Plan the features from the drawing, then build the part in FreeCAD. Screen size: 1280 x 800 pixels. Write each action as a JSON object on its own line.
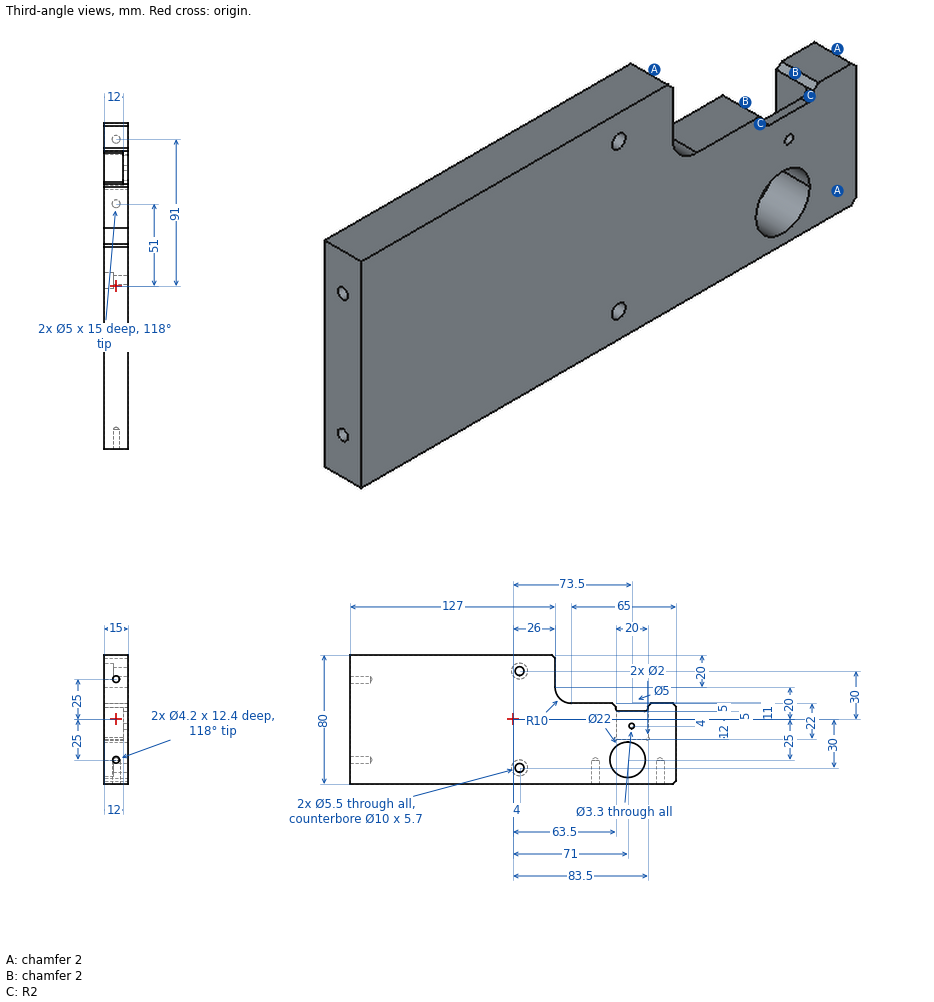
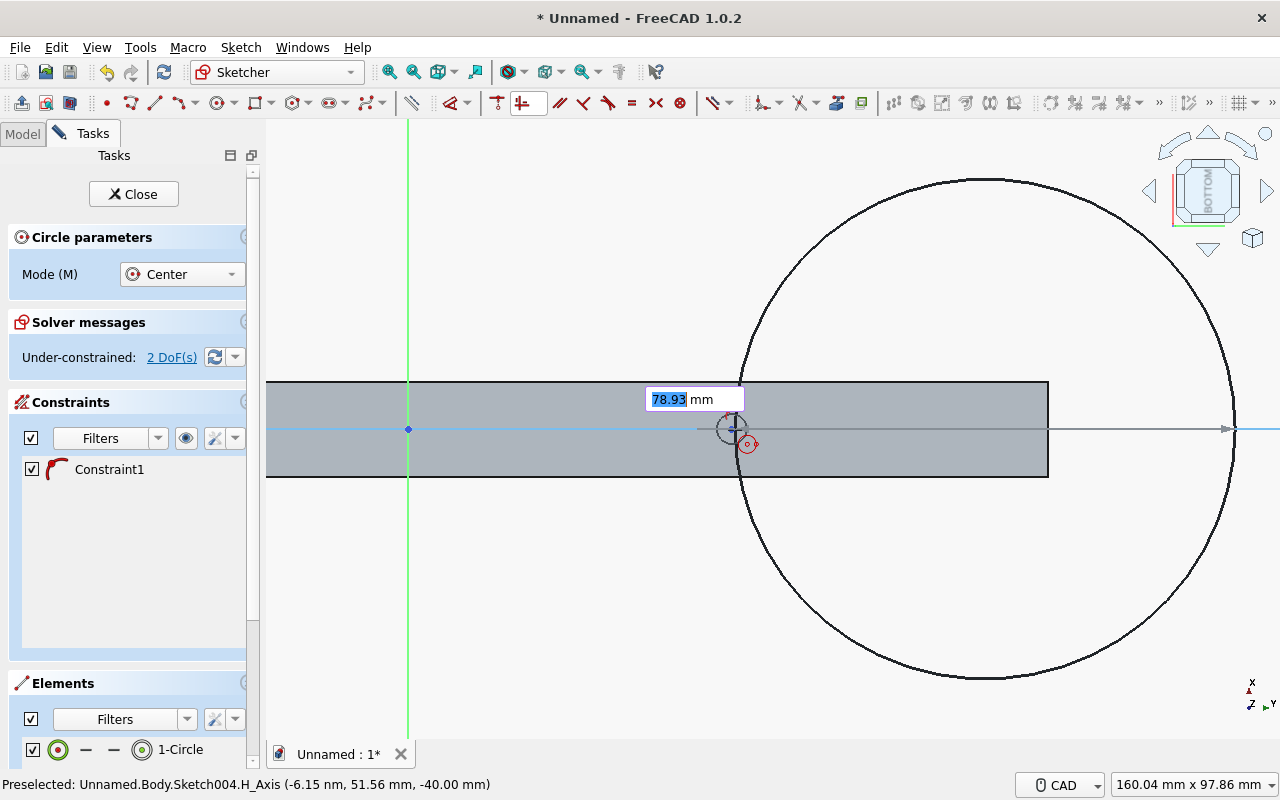
{"action": "scroll", "coordinate": [996, 418], "scroll_direction": "up", "scroll_amount": 2}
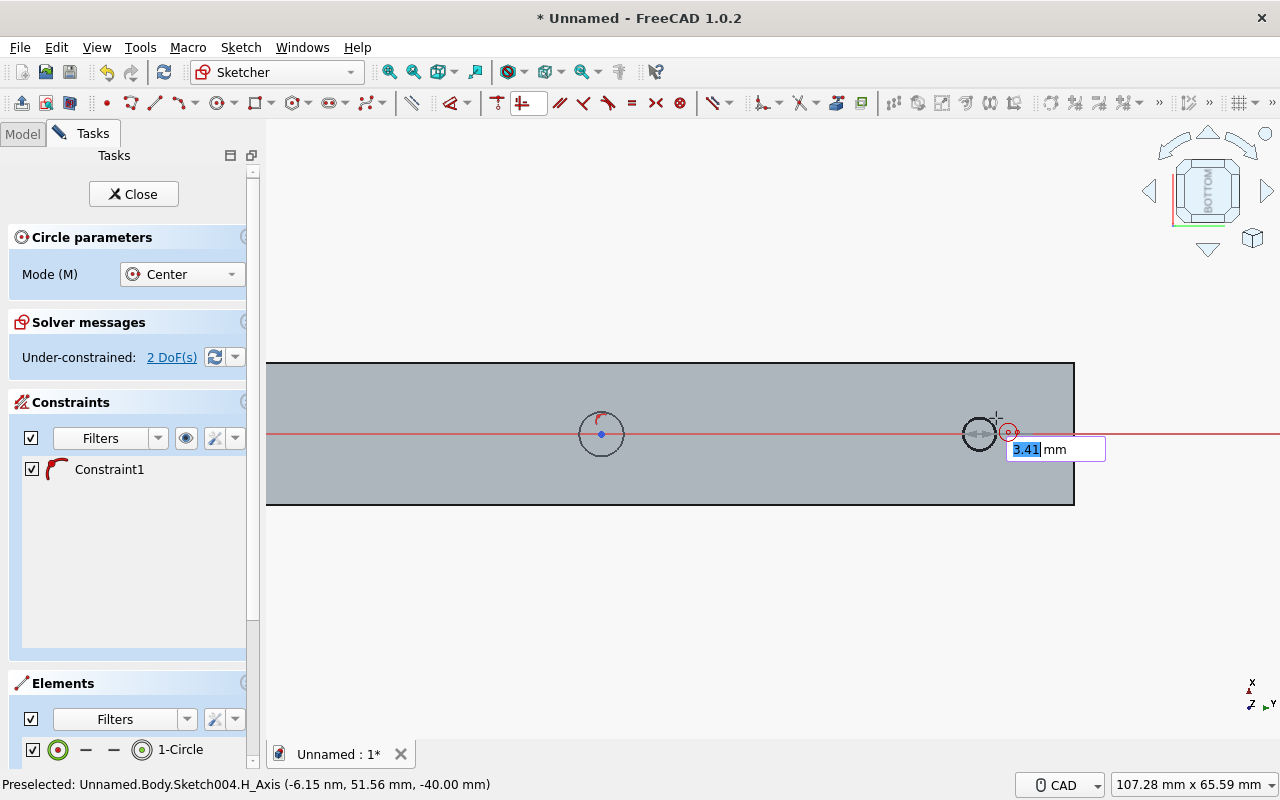
{"action": "left_click", "coordinate": [996, 418]}
{"action": "key", "text": "Escape"}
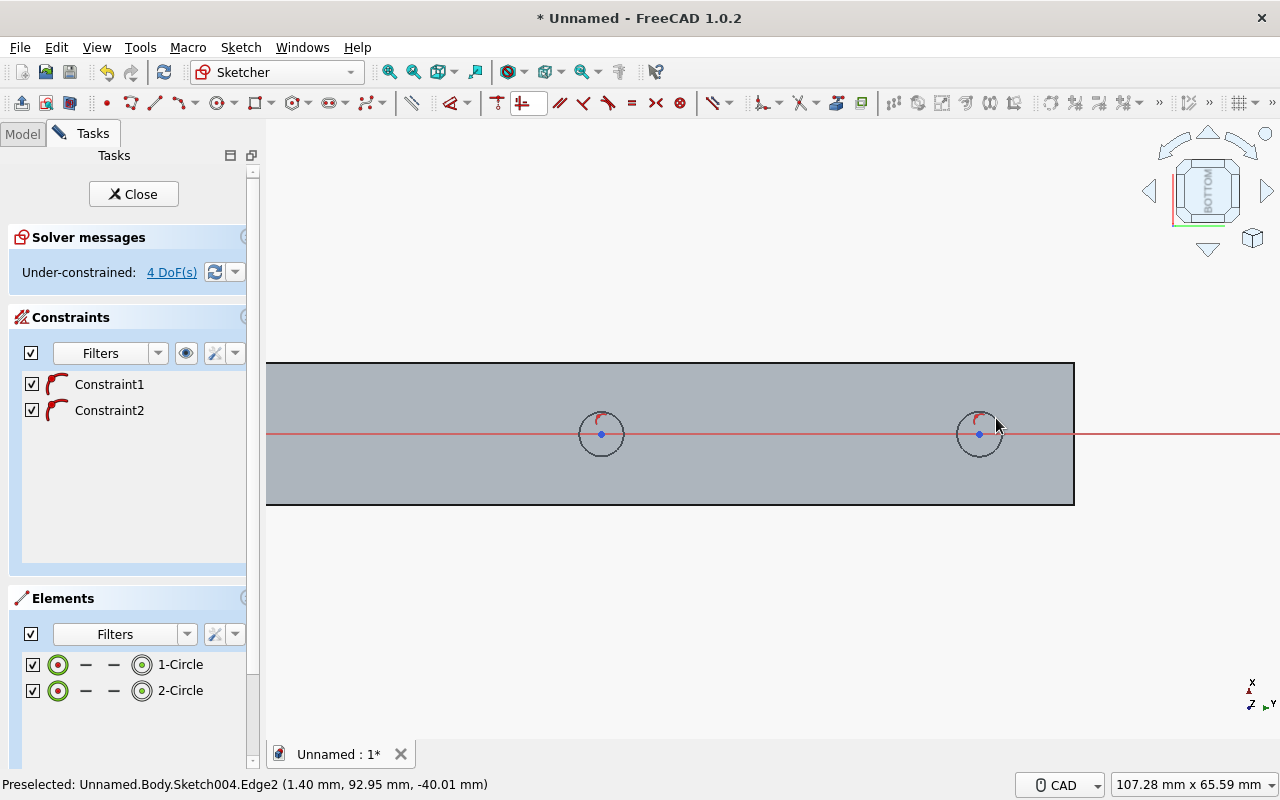
{"action": "left_click", "coordinate": [617, 419]}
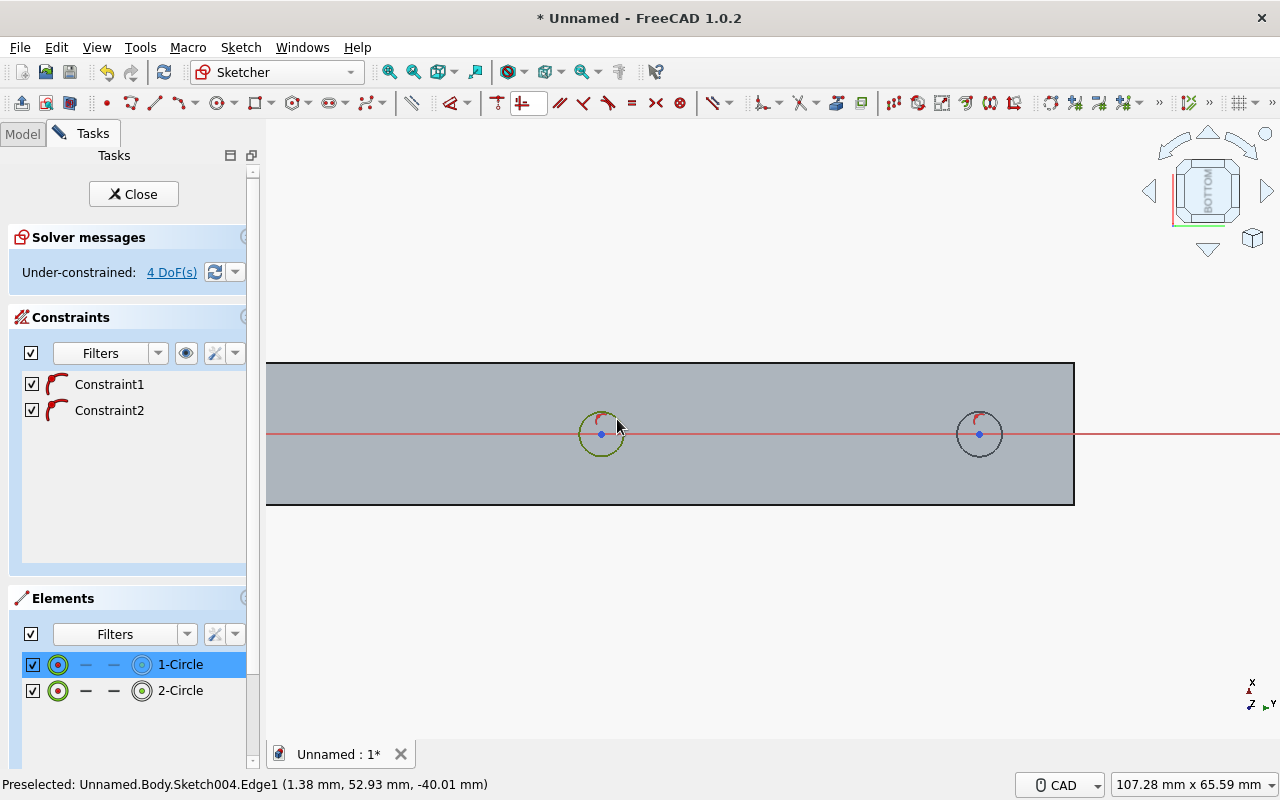
{"action": "left_click", "coordinate": [995, 418]}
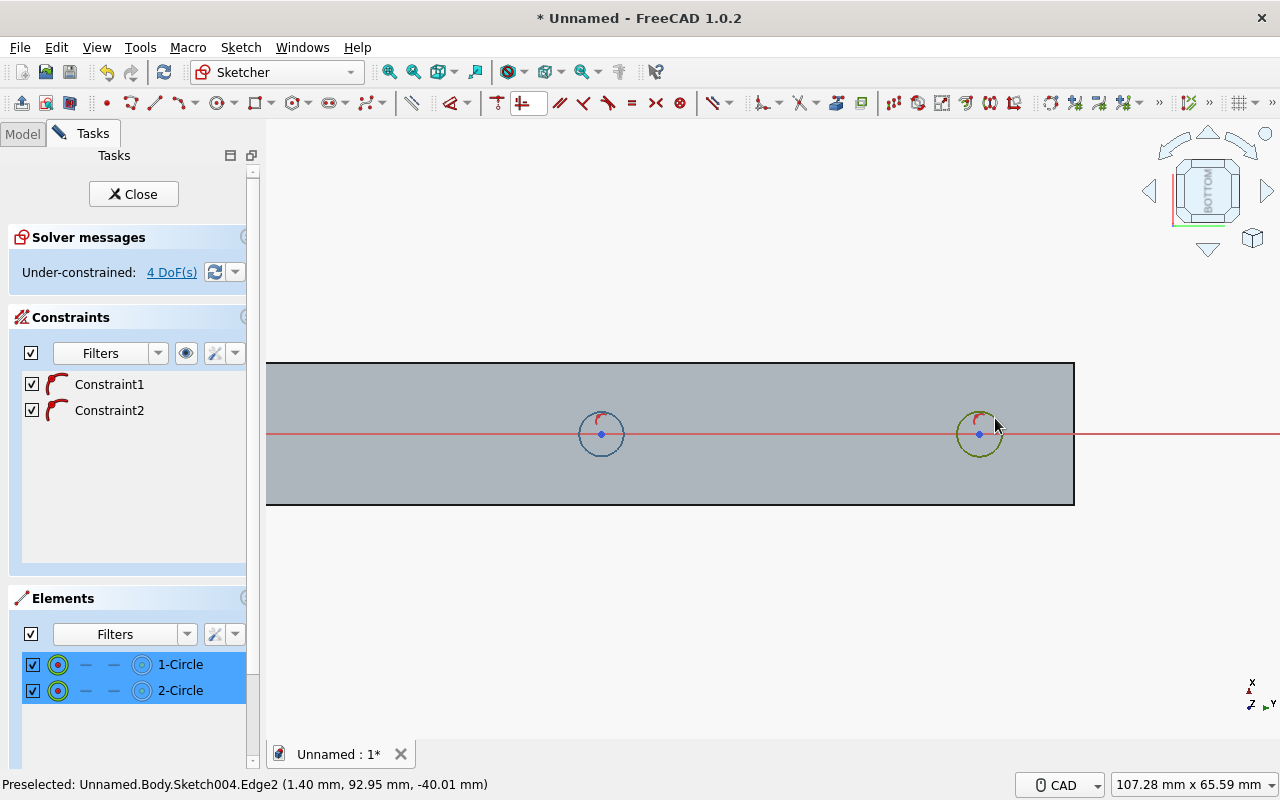
{"action": "left_click", "coordinate": [632, 104]}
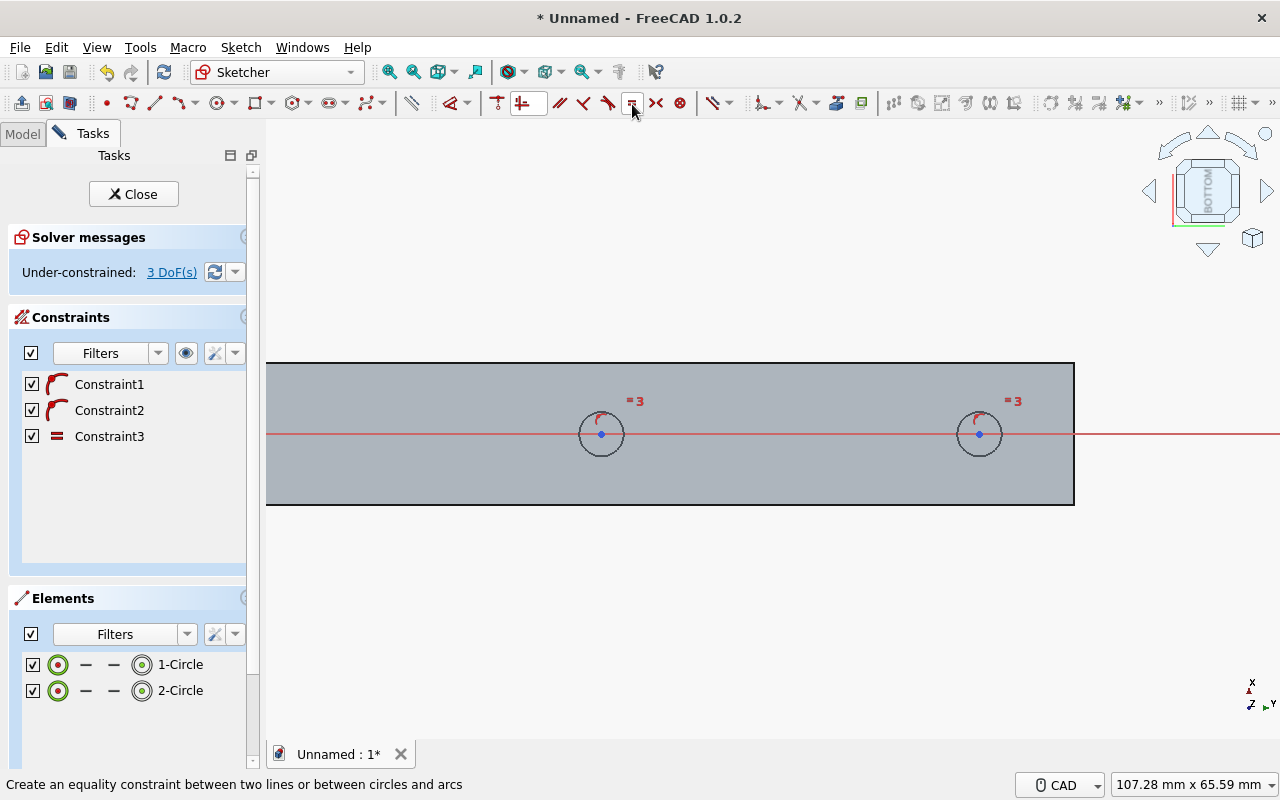
{"action": "left_click", "coordinate": [450, 104]}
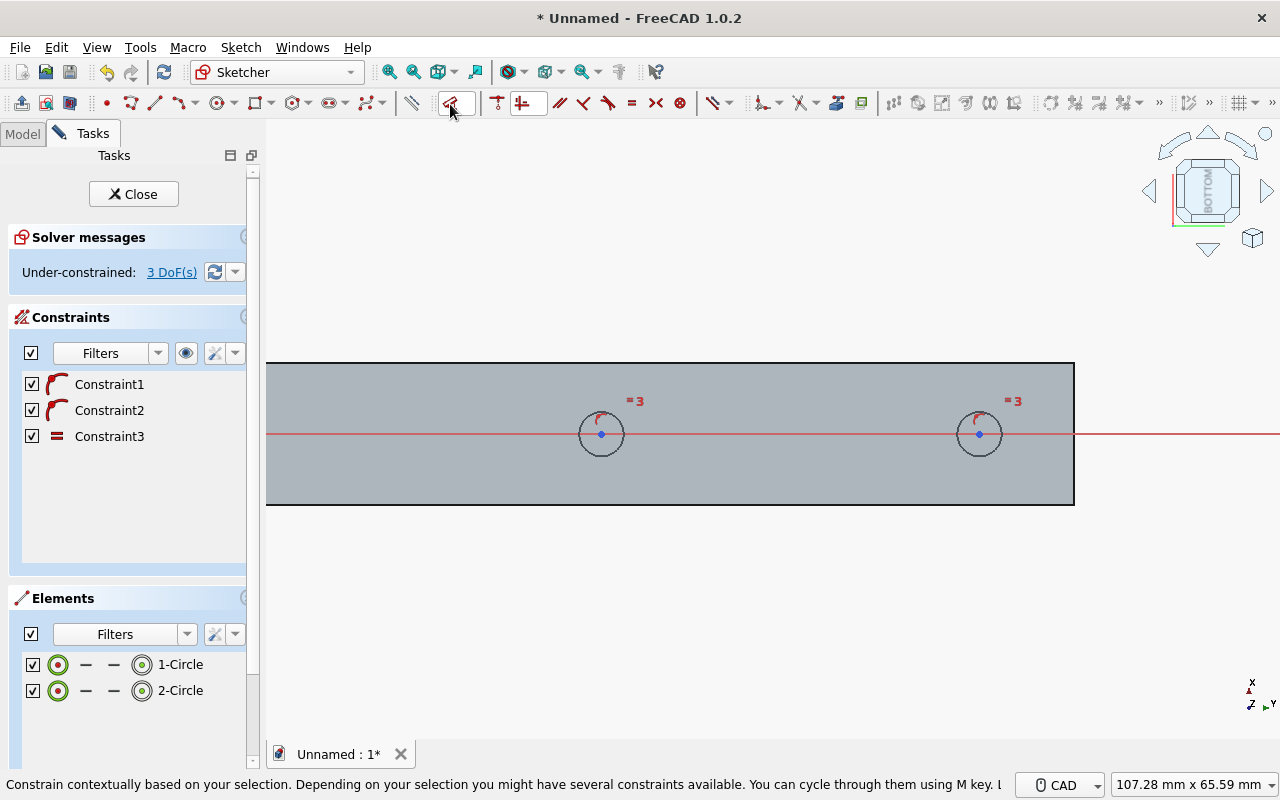
{"action": "left_click", "coordinate": [617, 419]}
{"action": "left_click", "coordinate": [640, 397]}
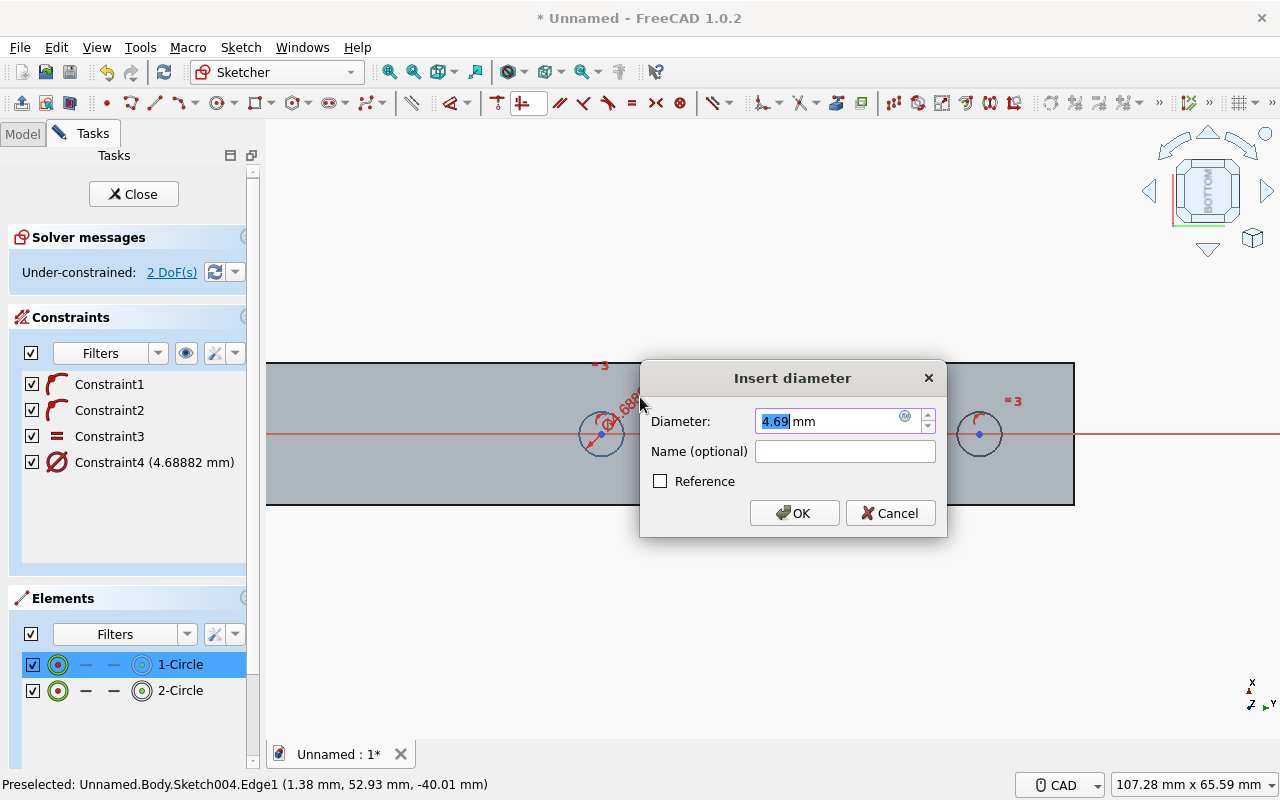
{"action": "type", "text": "5"}
{"action": "key", "text": "Return"}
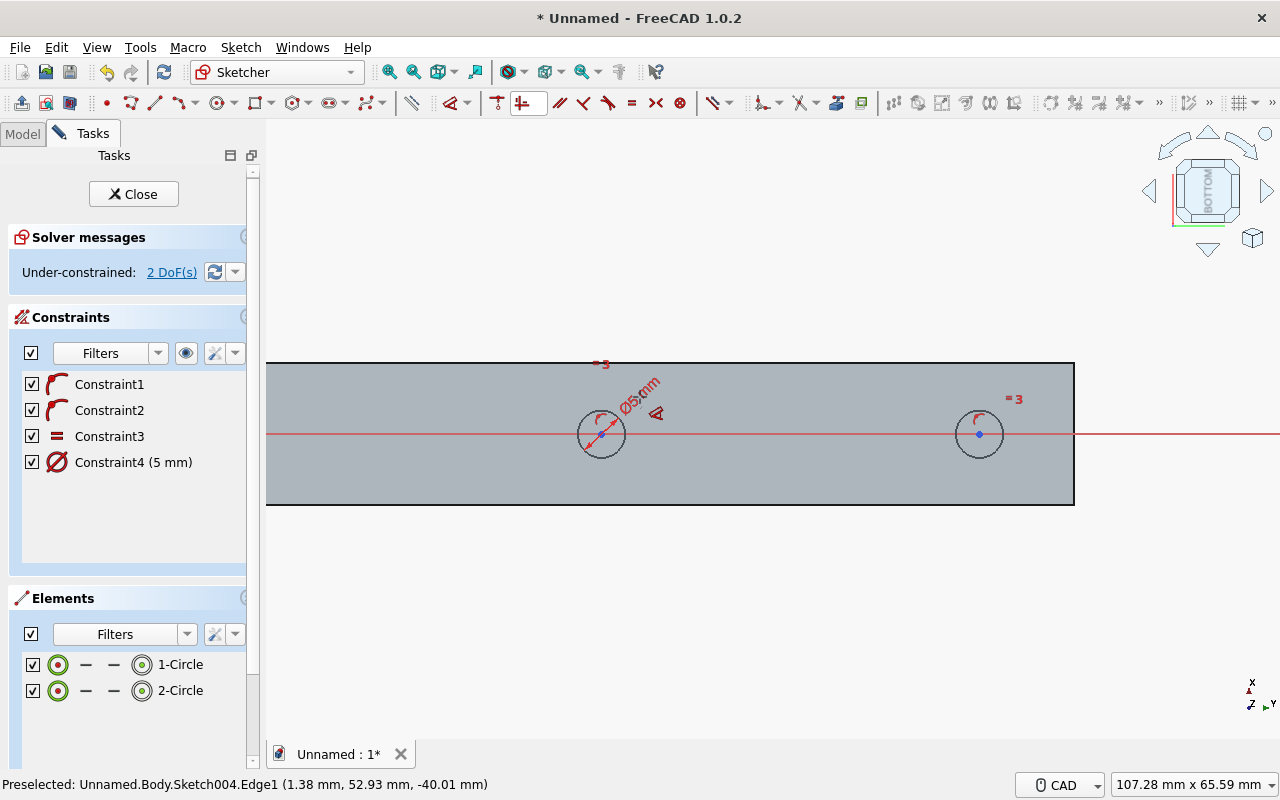
{"action": "left_click", "coordinate": [602, 434]}
{"action": "left_click", "coordinate": [448, 468]}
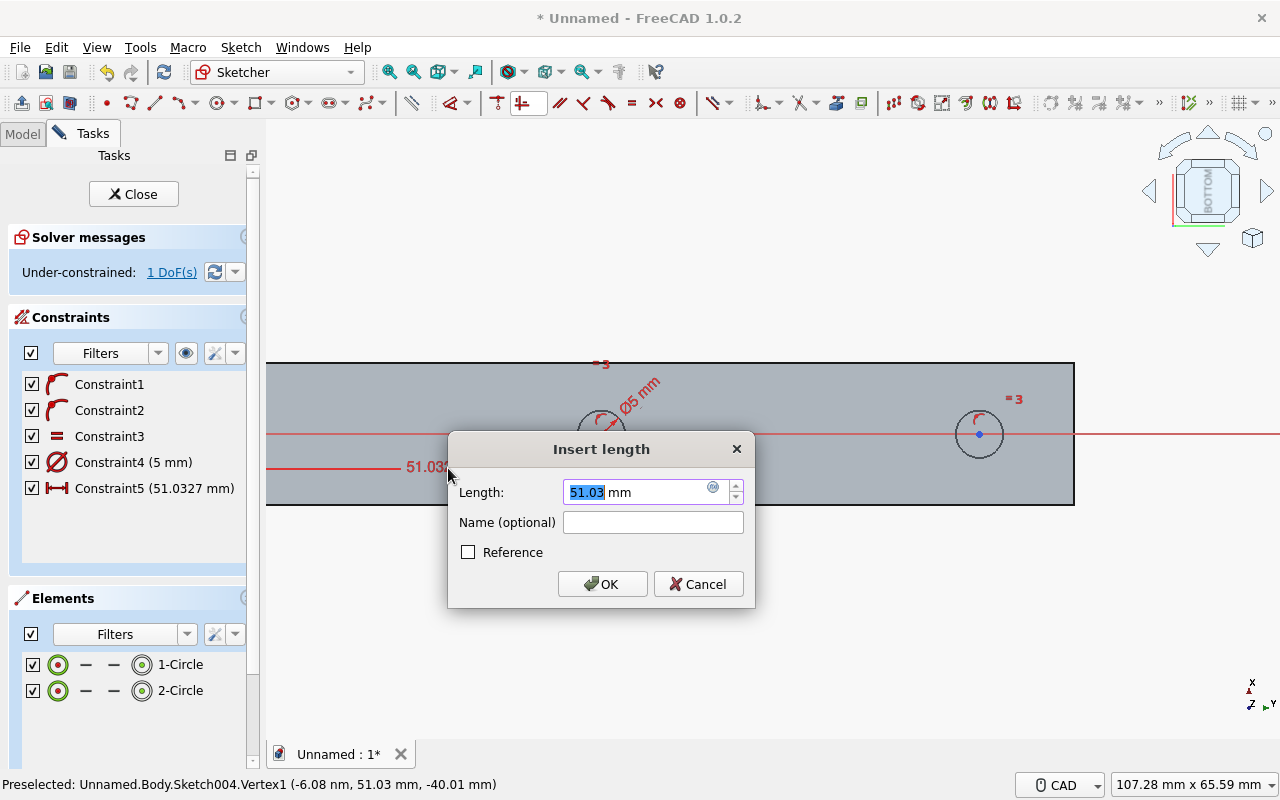
{"action": "type", "text": "51"}
{"action": "key", "text": "Return"}